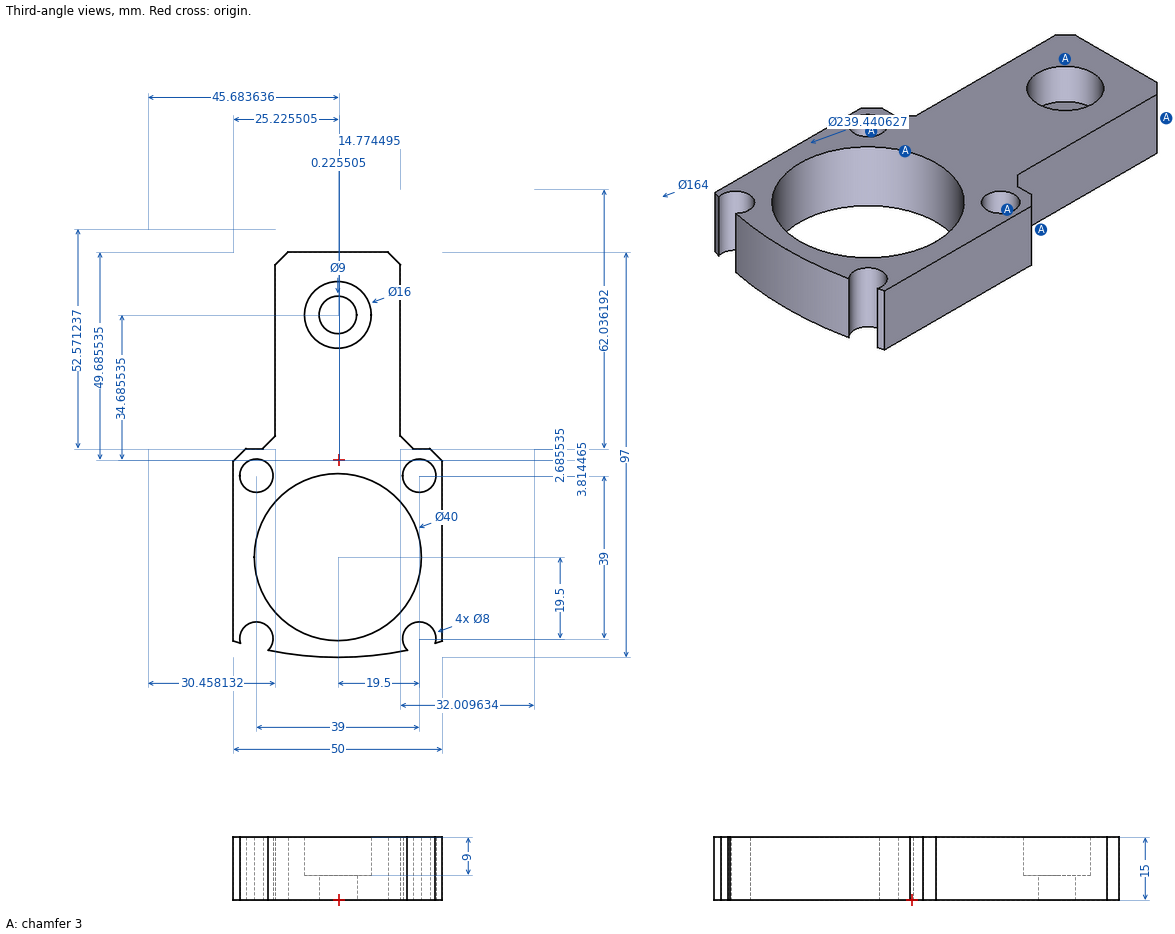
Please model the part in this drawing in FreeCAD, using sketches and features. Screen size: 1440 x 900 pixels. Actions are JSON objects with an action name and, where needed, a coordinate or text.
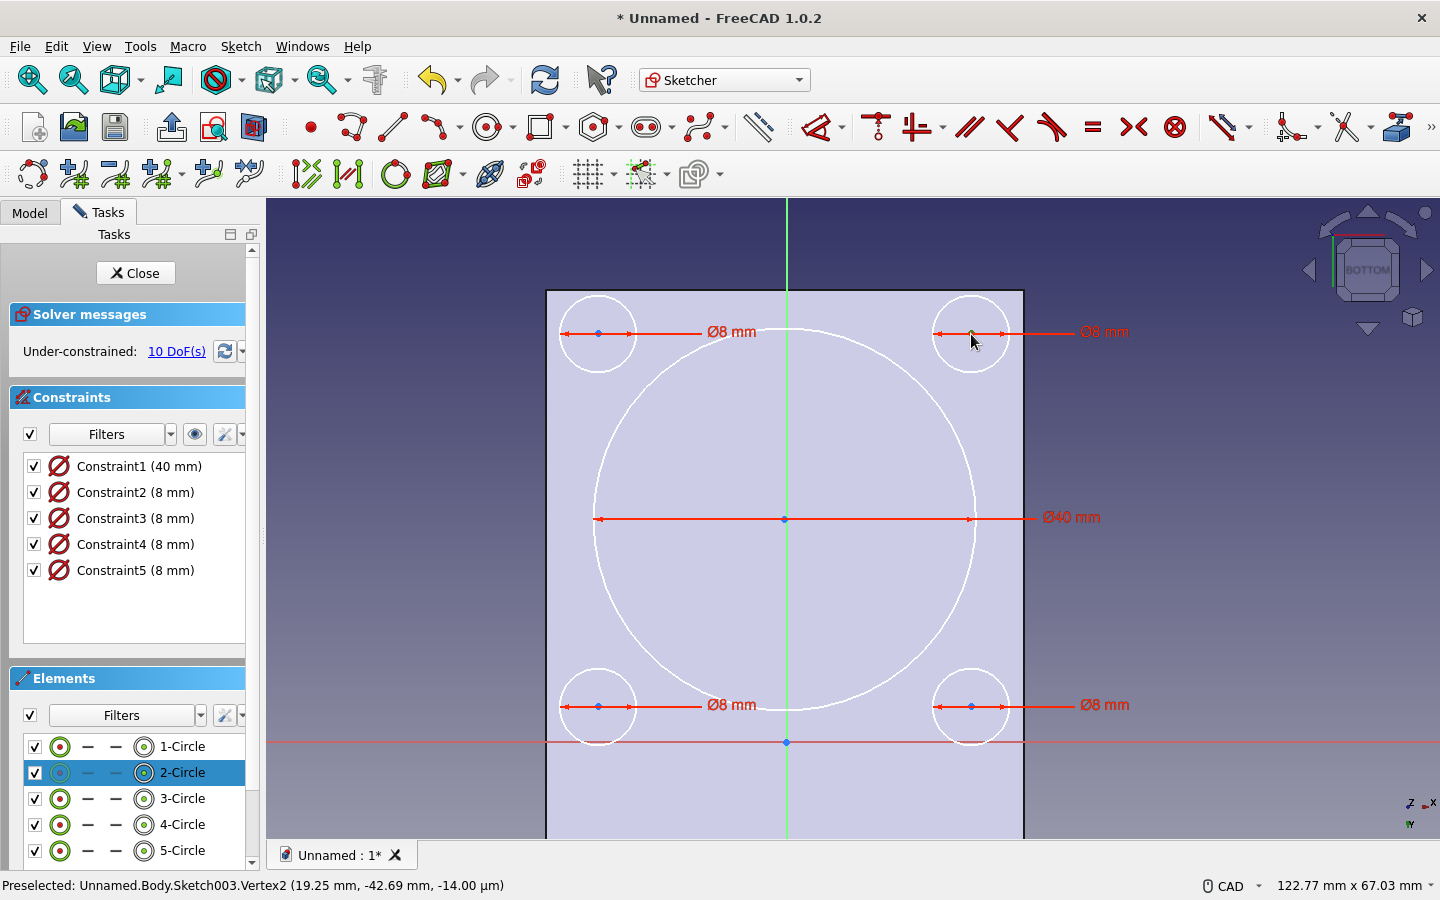
{"action": "left_click", "coordinate": [971, 707]}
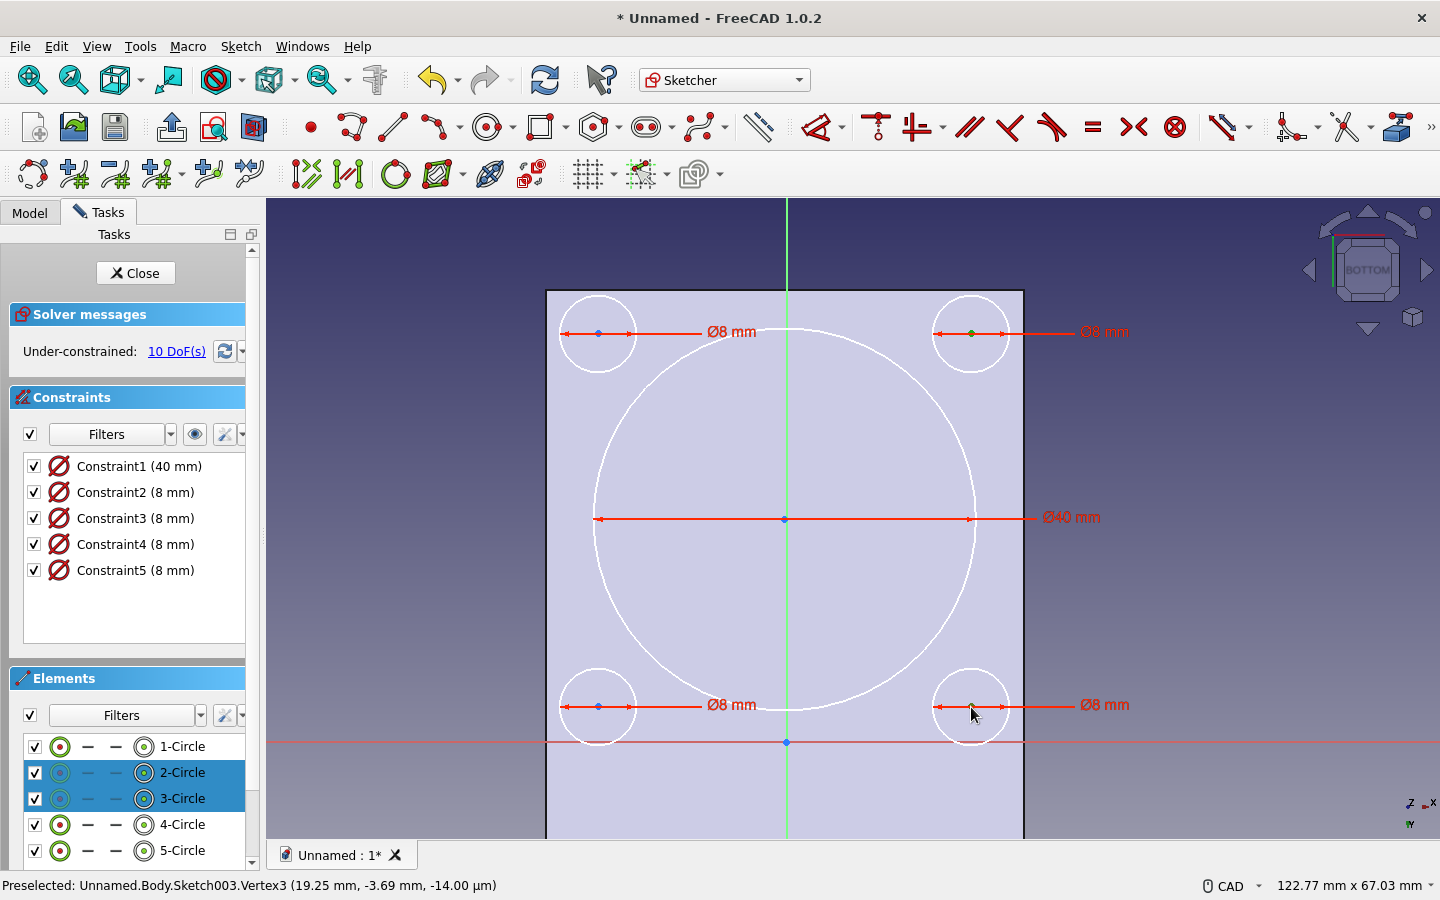
{"action": "key", "text": "v"}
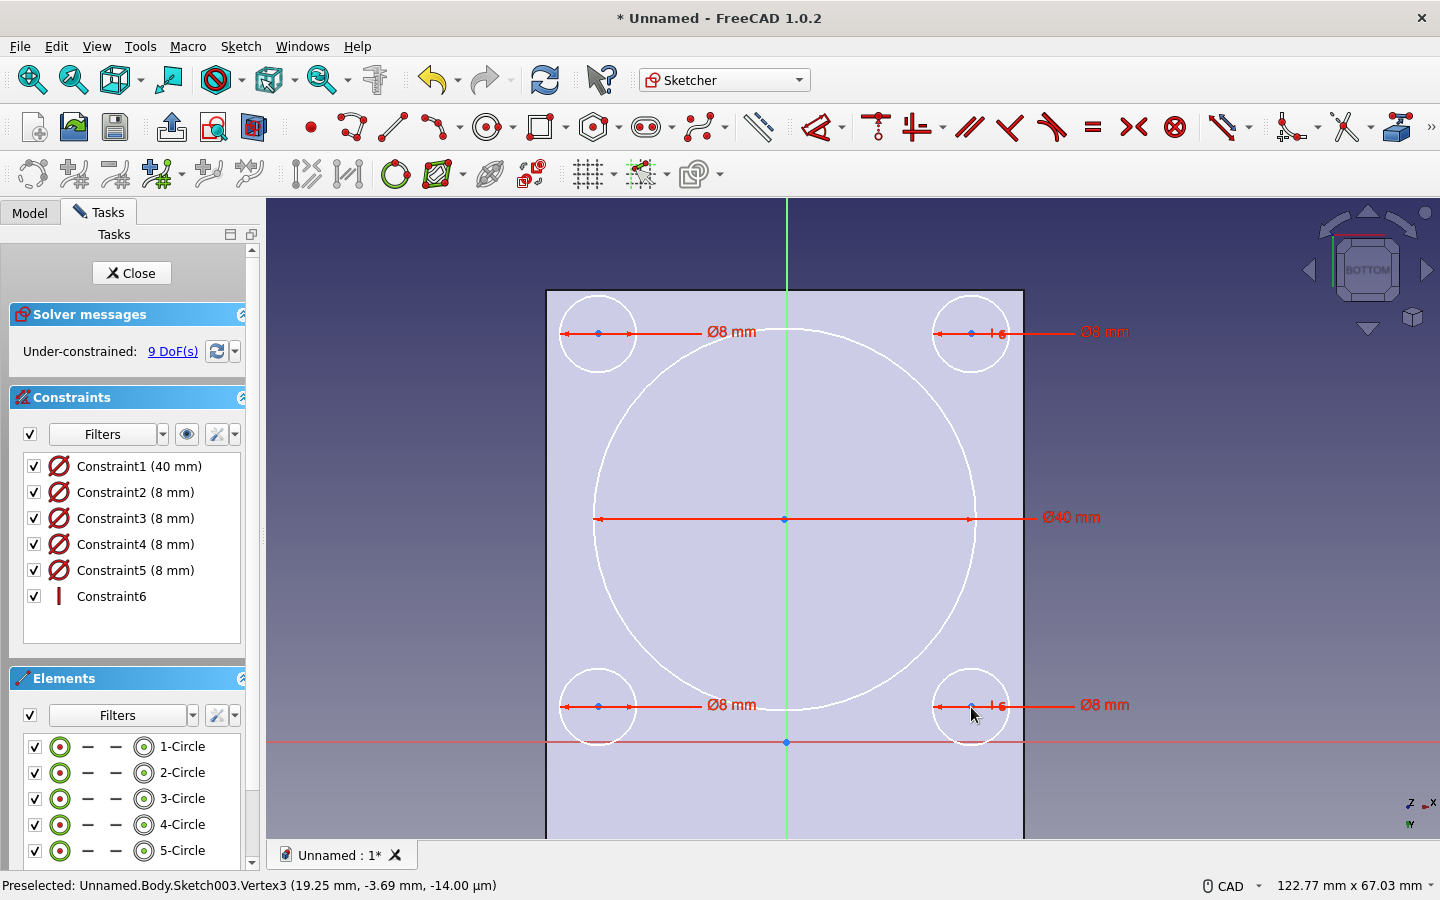
{"action": "left_click", "coordinate": [971, 707]}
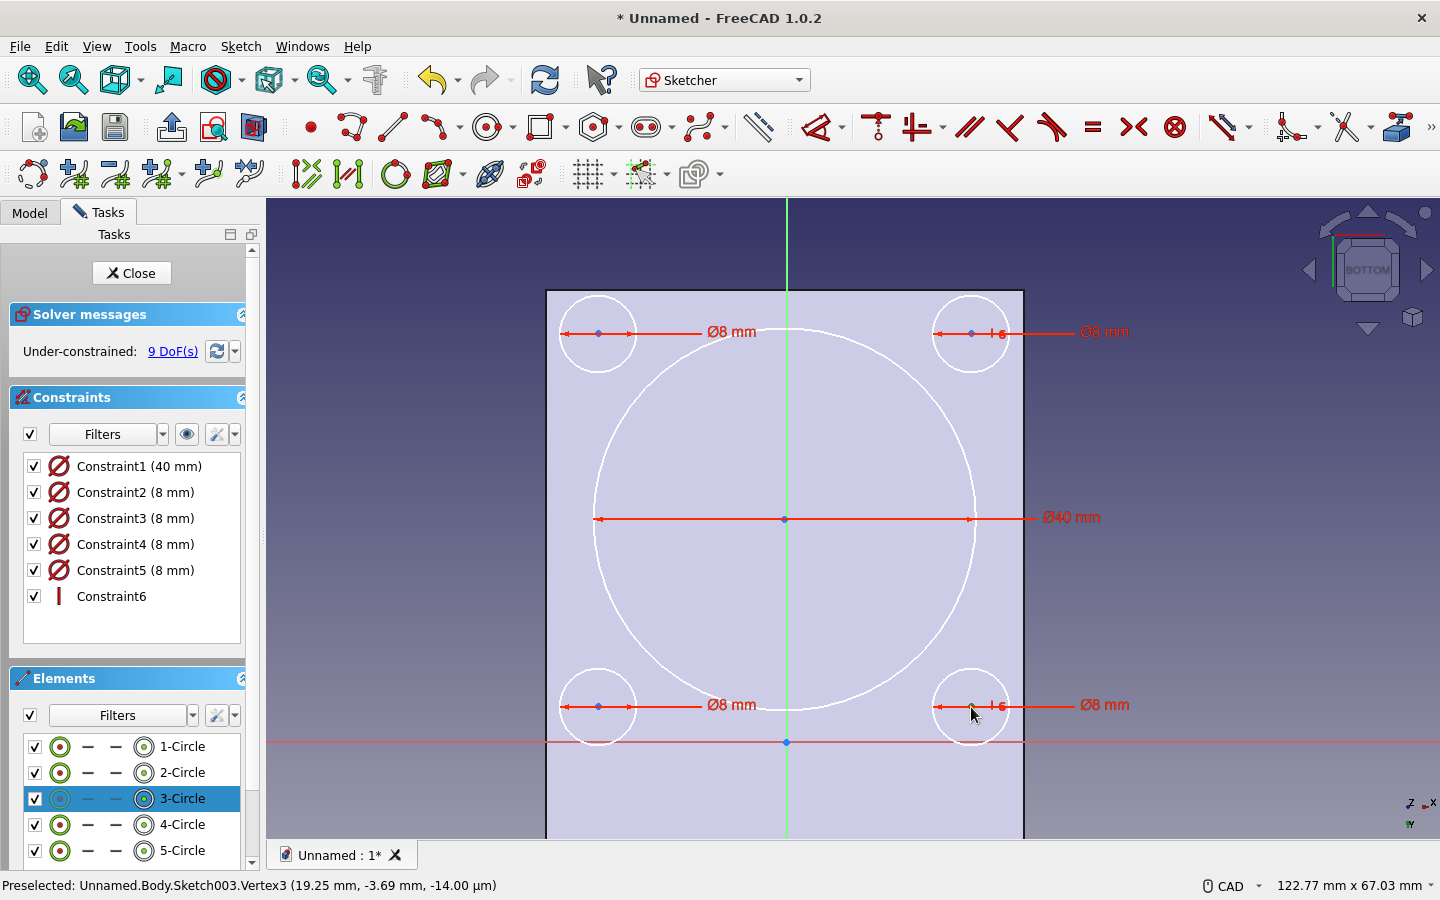
{"action": "left_click", "coordinate": [598, 707]}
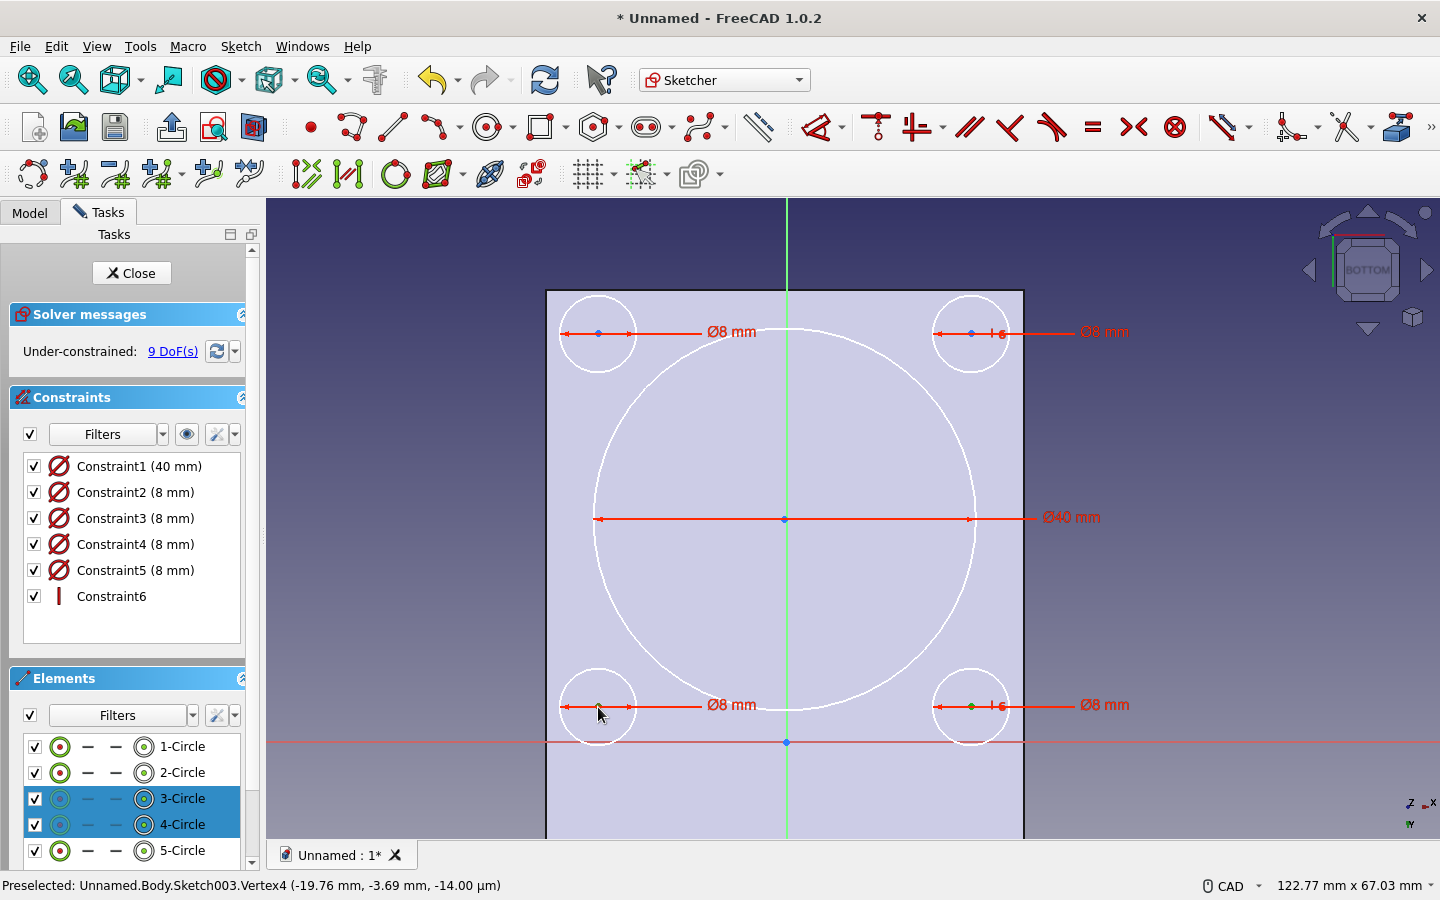
{"action": "left_click", "coordinate": [942, 128]}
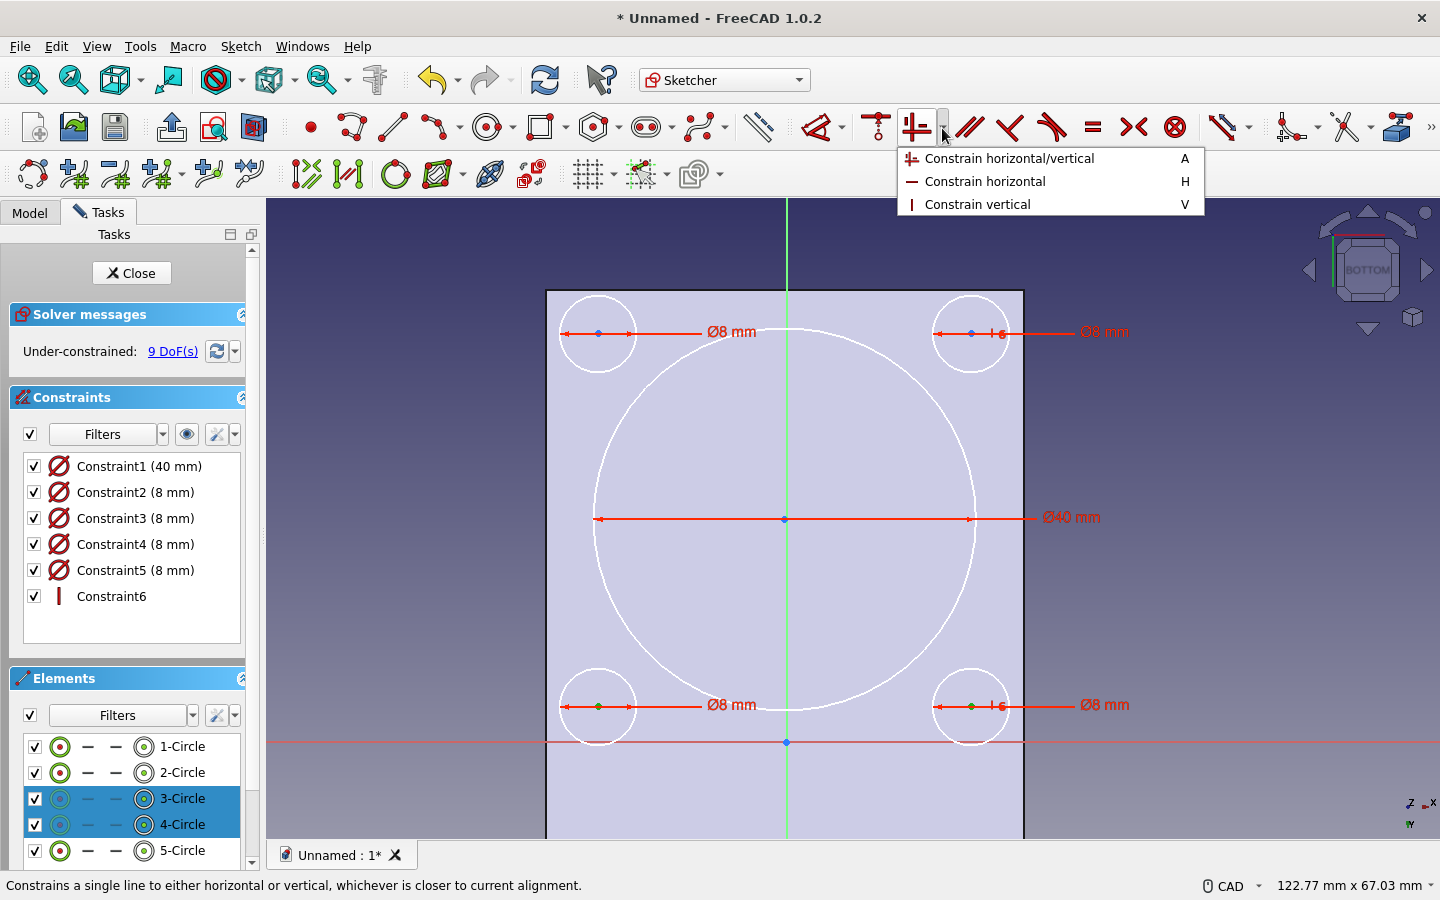
{"action": "left_click", "coordinate": [1051, 182]}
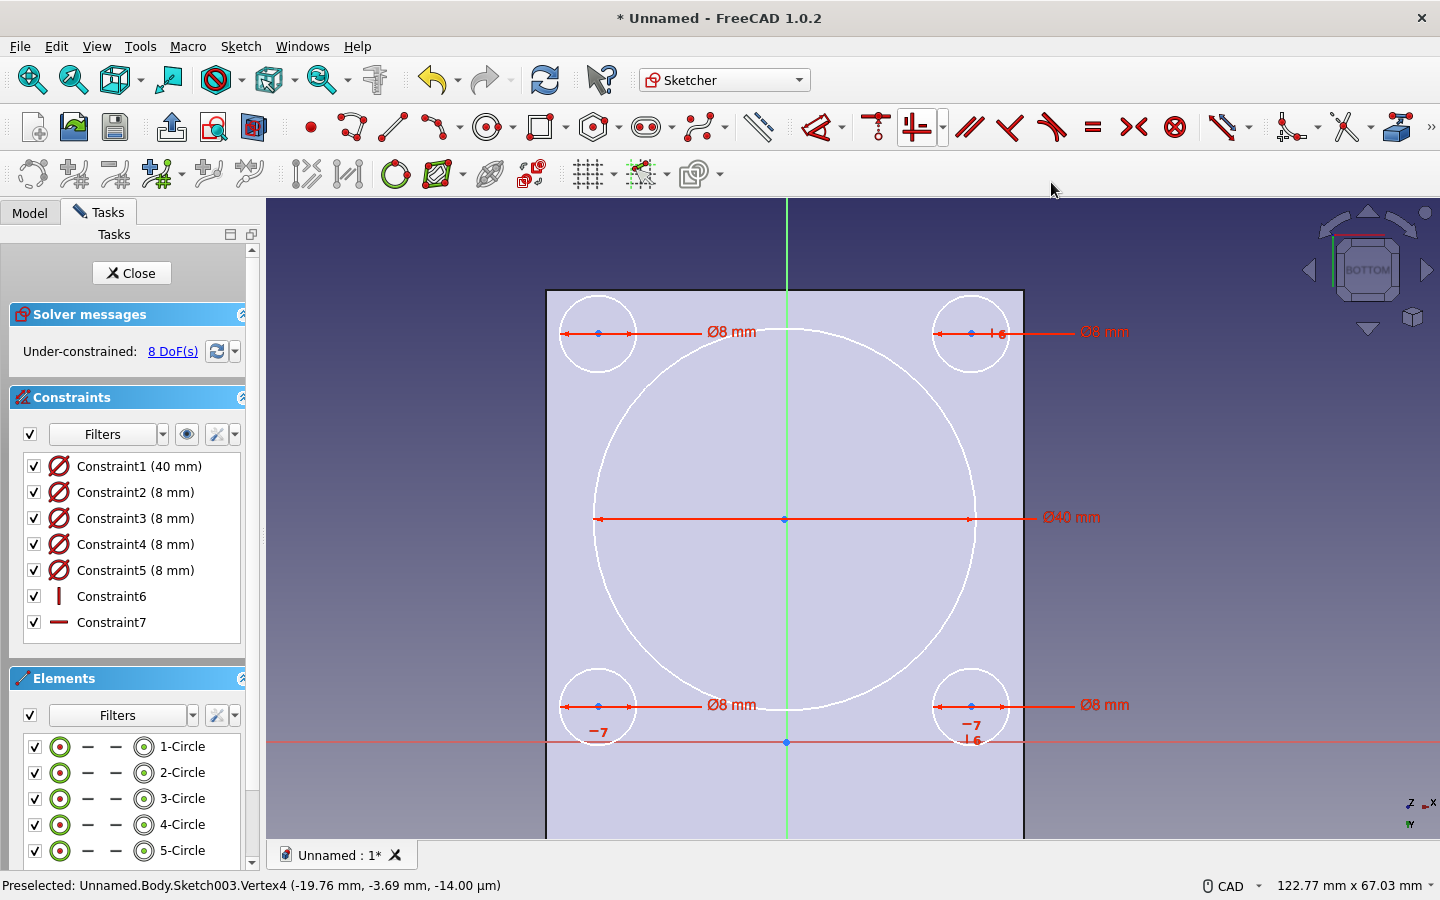
{"action": "left_click", "coordinate": [598, 707]}